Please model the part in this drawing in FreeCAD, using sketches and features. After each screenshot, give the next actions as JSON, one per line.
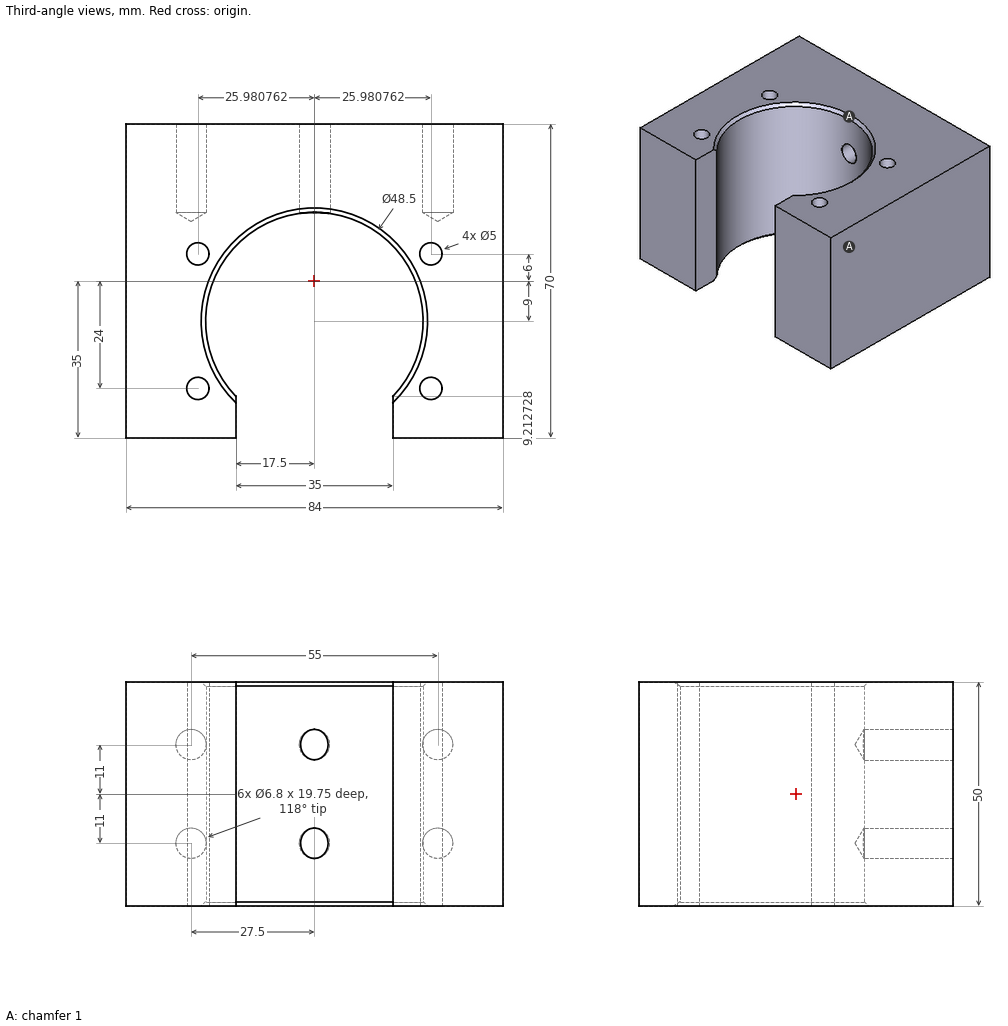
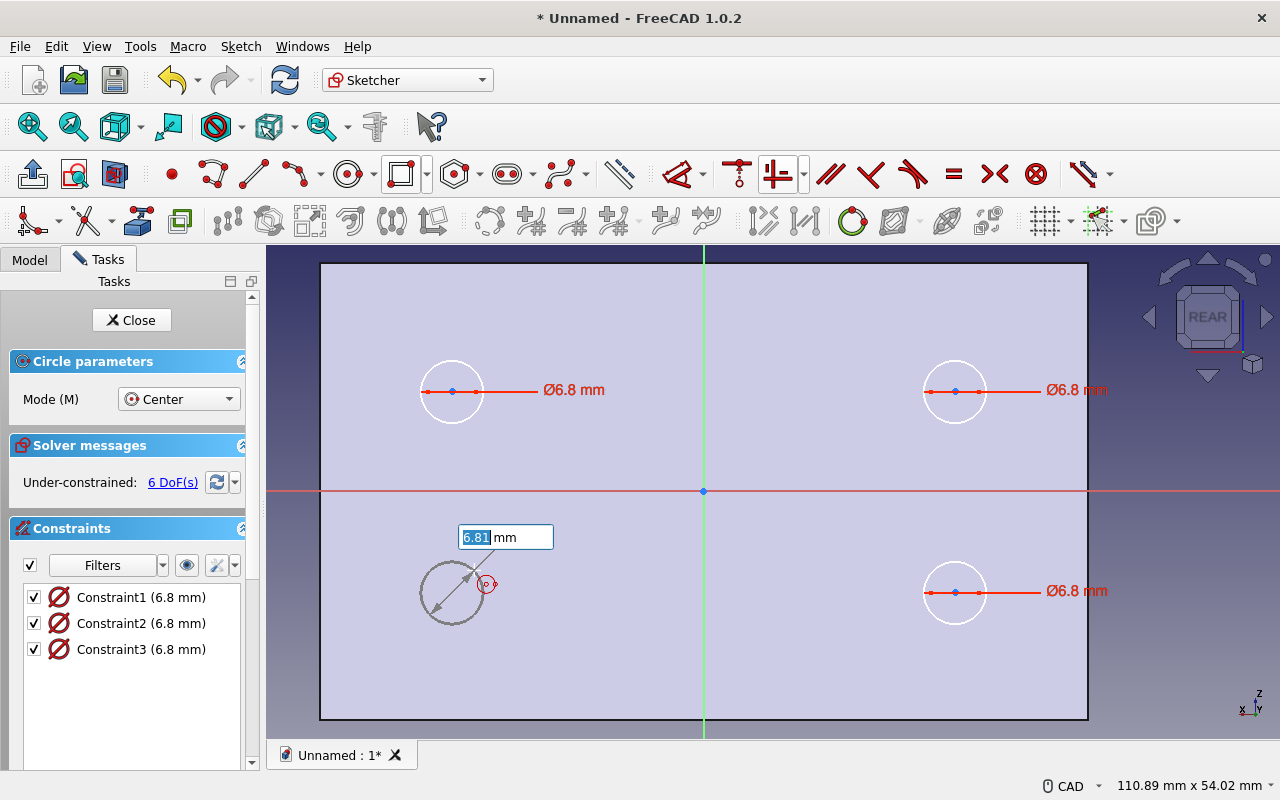
{"action": "type", "text": "6.8"}
{"action": "key", "text": "Return"}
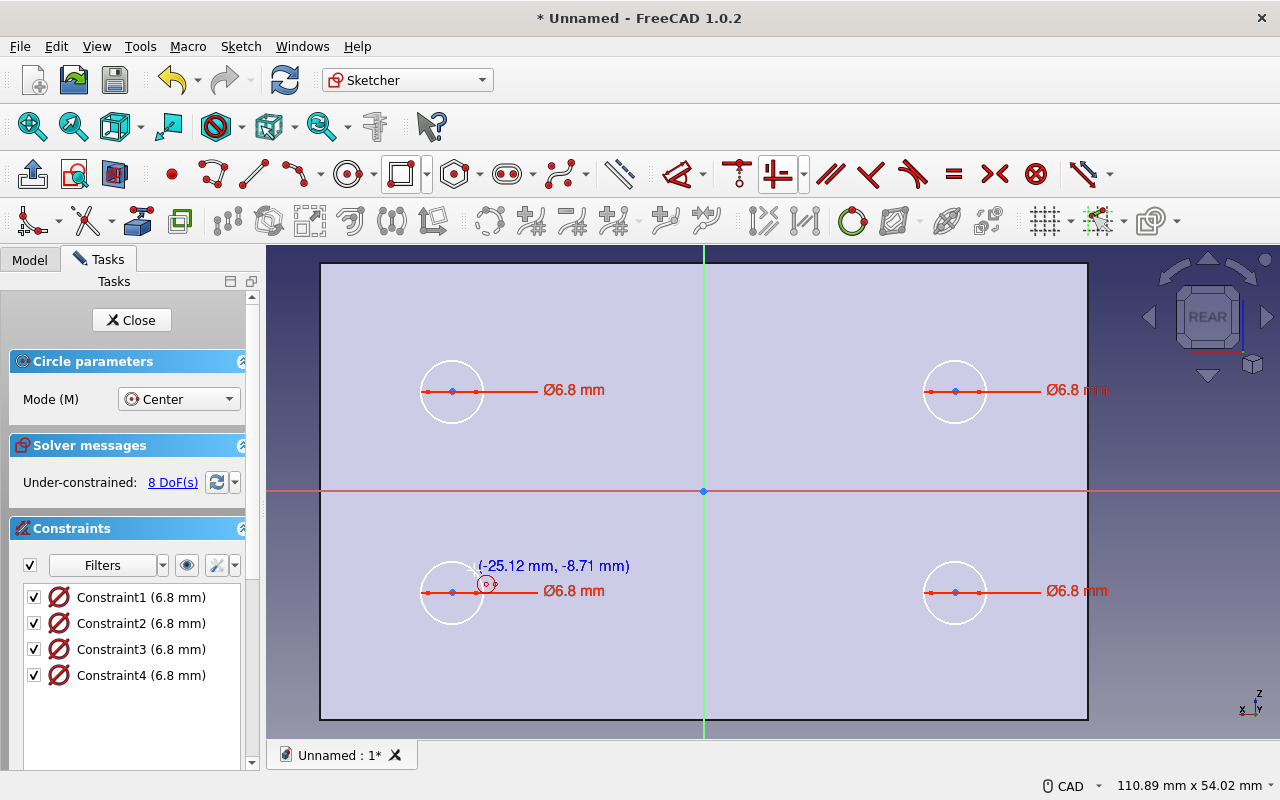
{"action": "left_click", "coordinate": [704, 592]}
{"action": "mouse_move", "coordinate": [726, 570]}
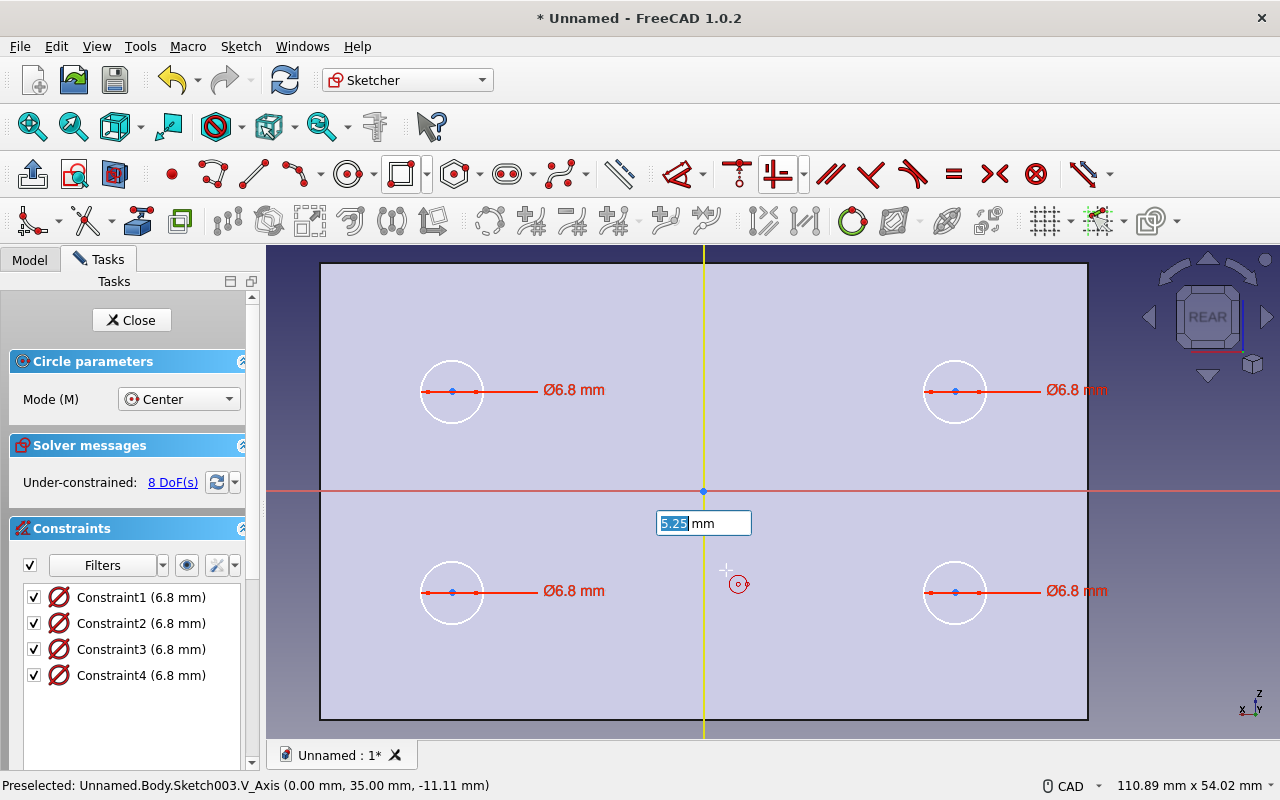
{"action": "type", "text": "6.8"}
{"action": "key", "text": "Return"}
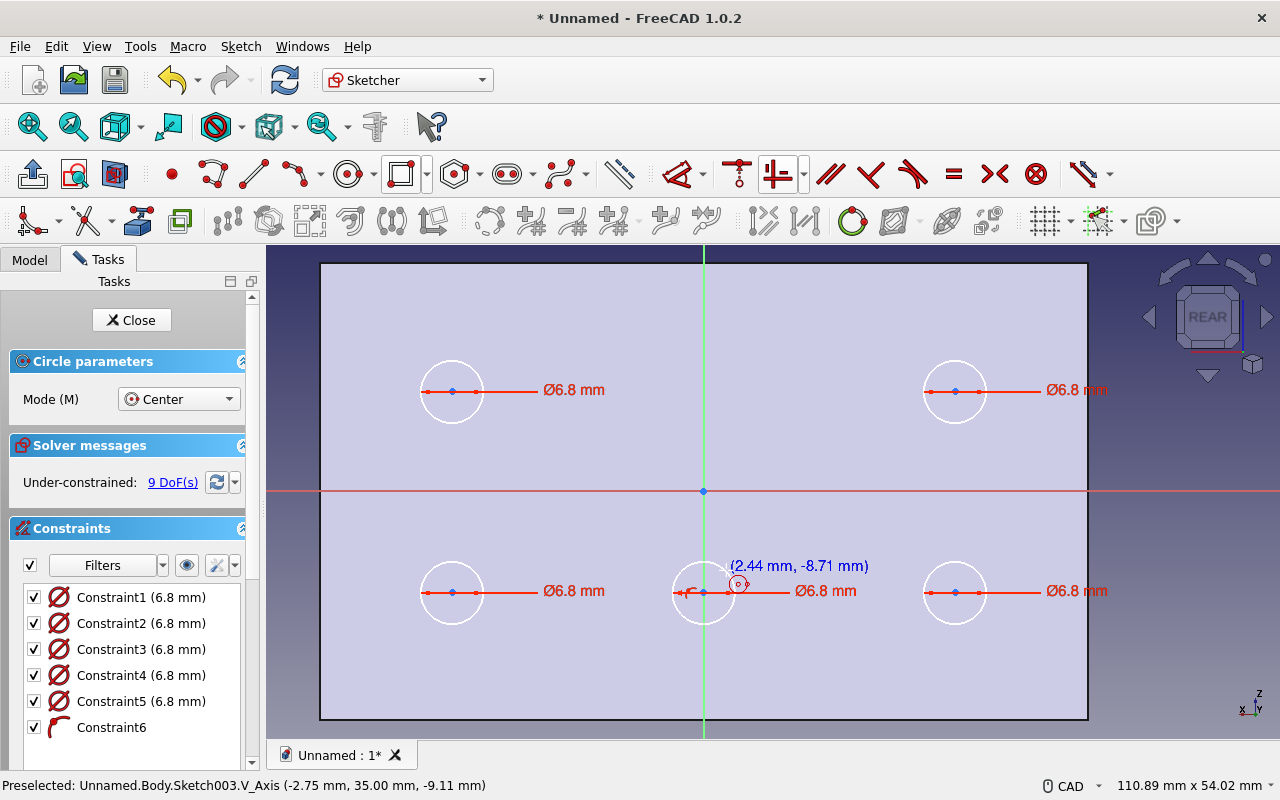
{"action": "left_click", "coordinate": [704, 391]}
{"action": "mouse_move", "coordinate": [726, 369]}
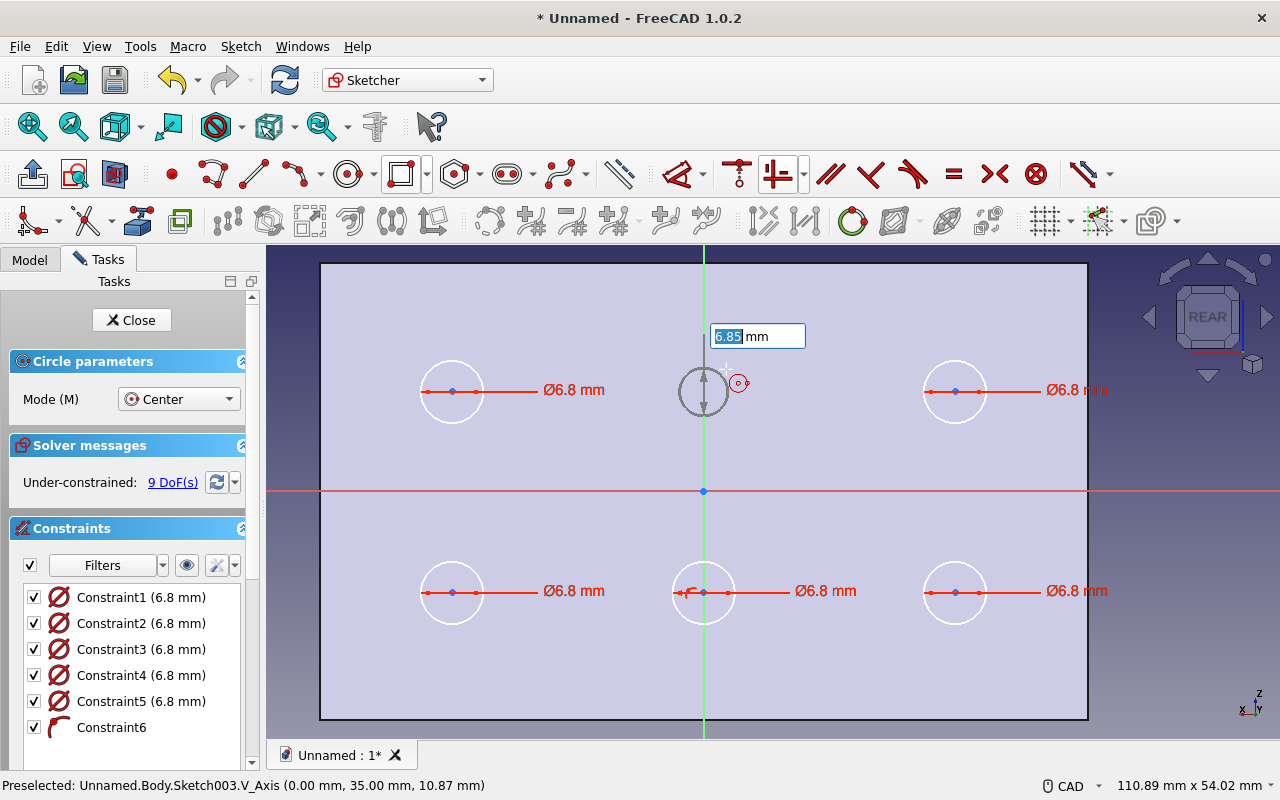
{"action": "type", "text": "6.8"}
{"action": "key", "text": "Return"}
{"action": "key", "text": "Escape"}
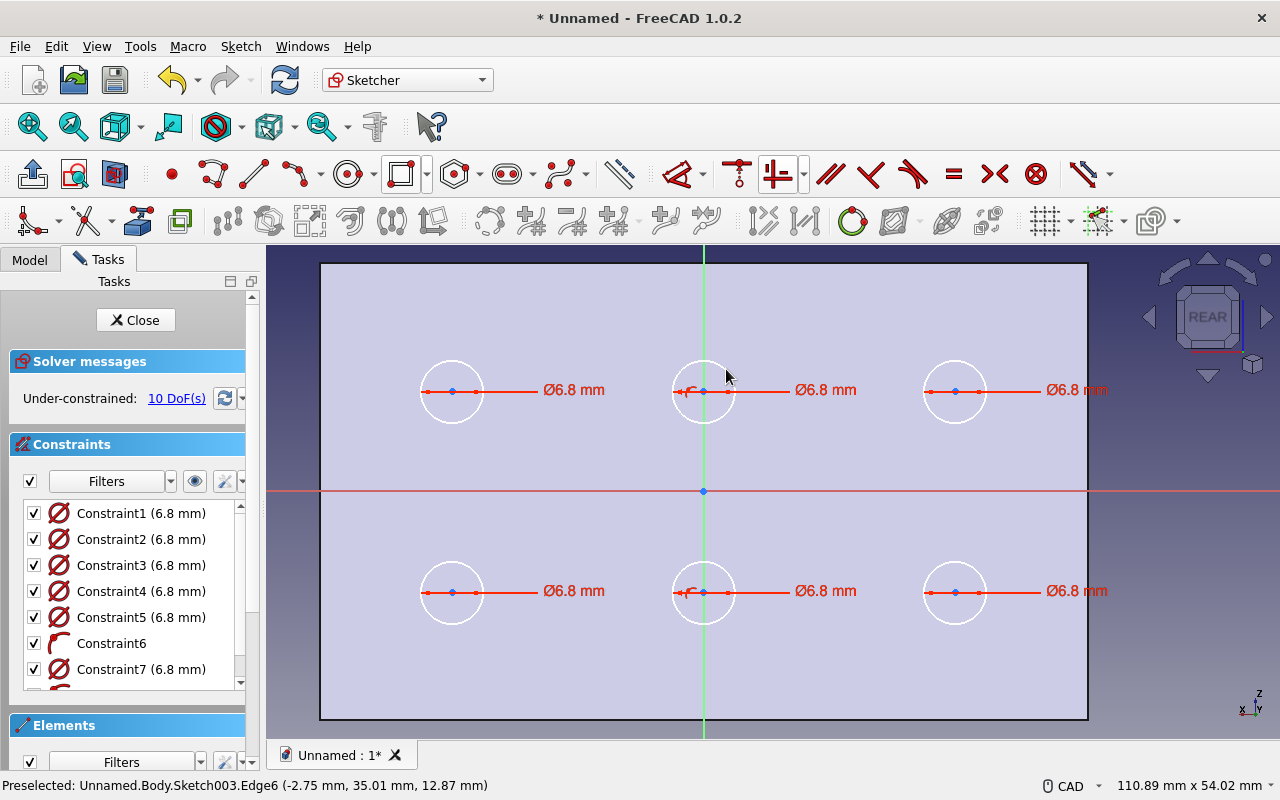
{"action": "left_click", "coordinate": [955, 593]}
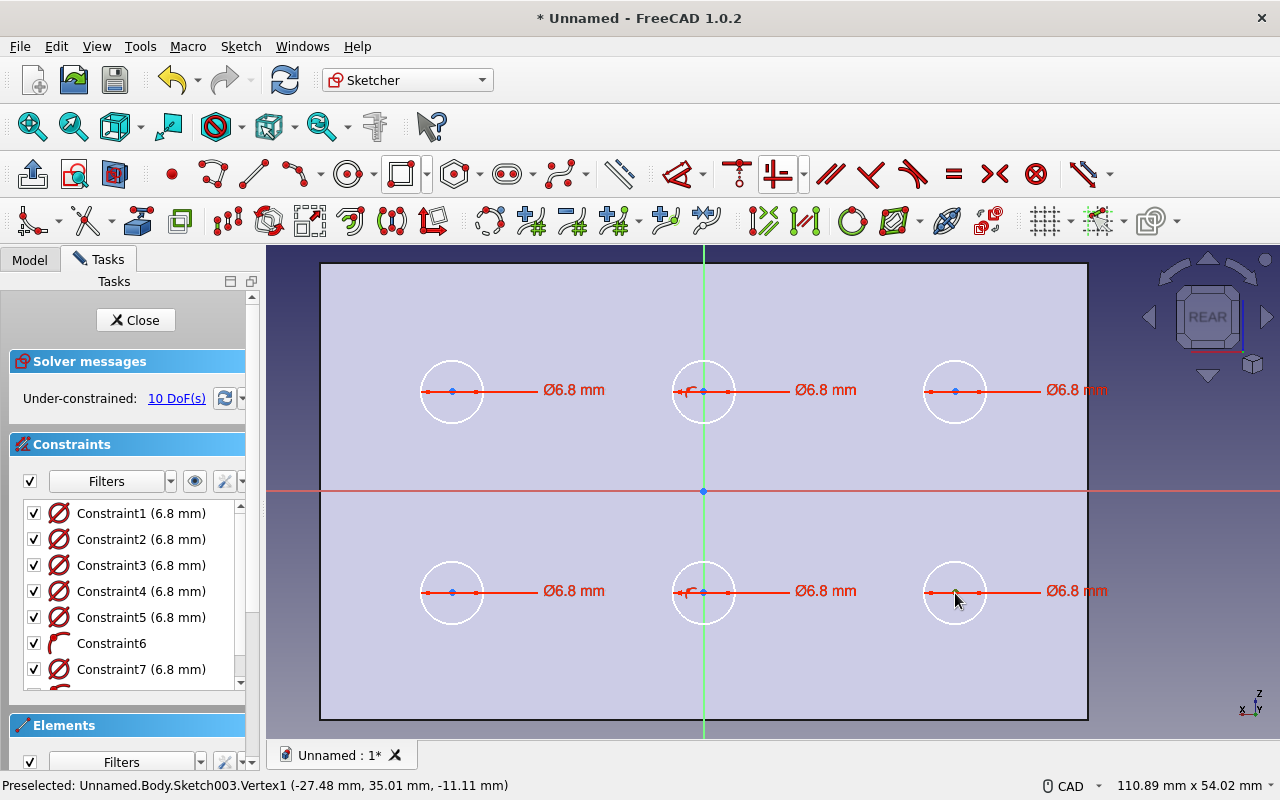
{"action": "left_click", "coordinate": [955, 392]}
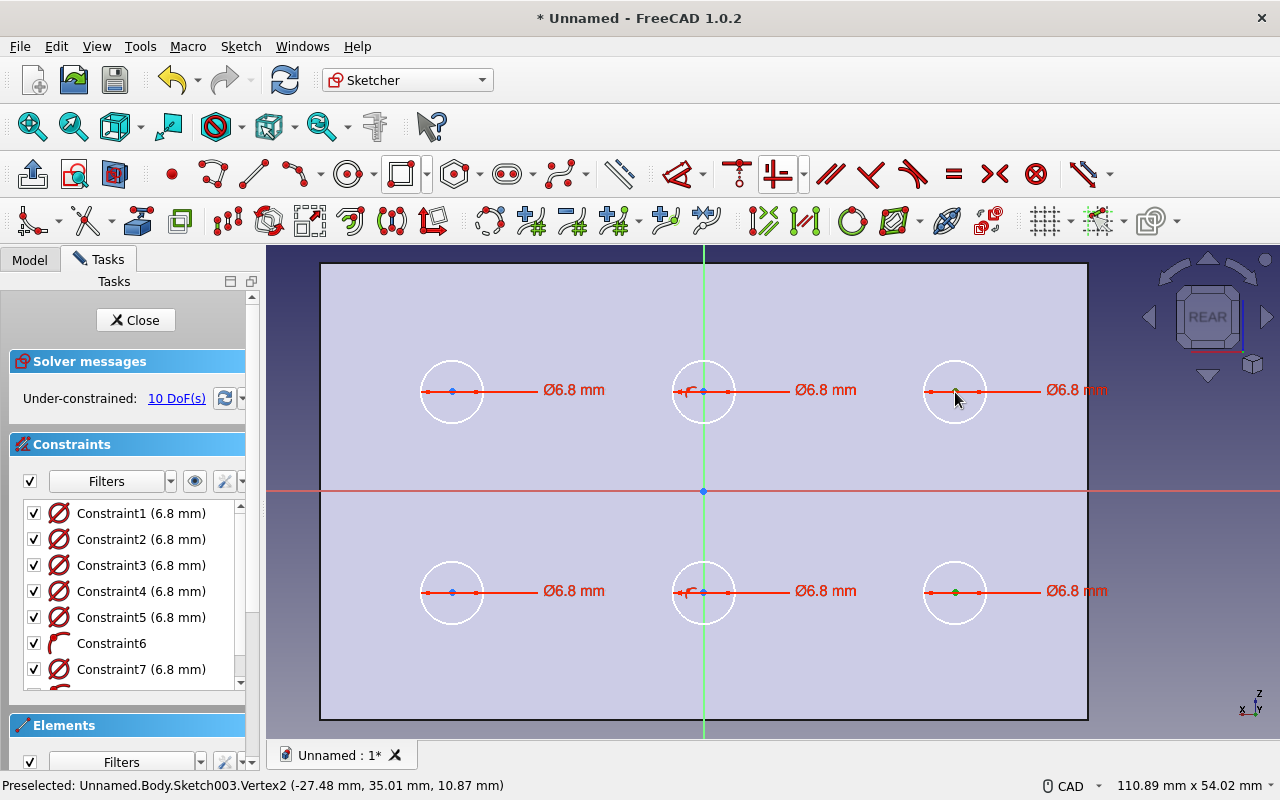
{"action": "key", "text": "v"}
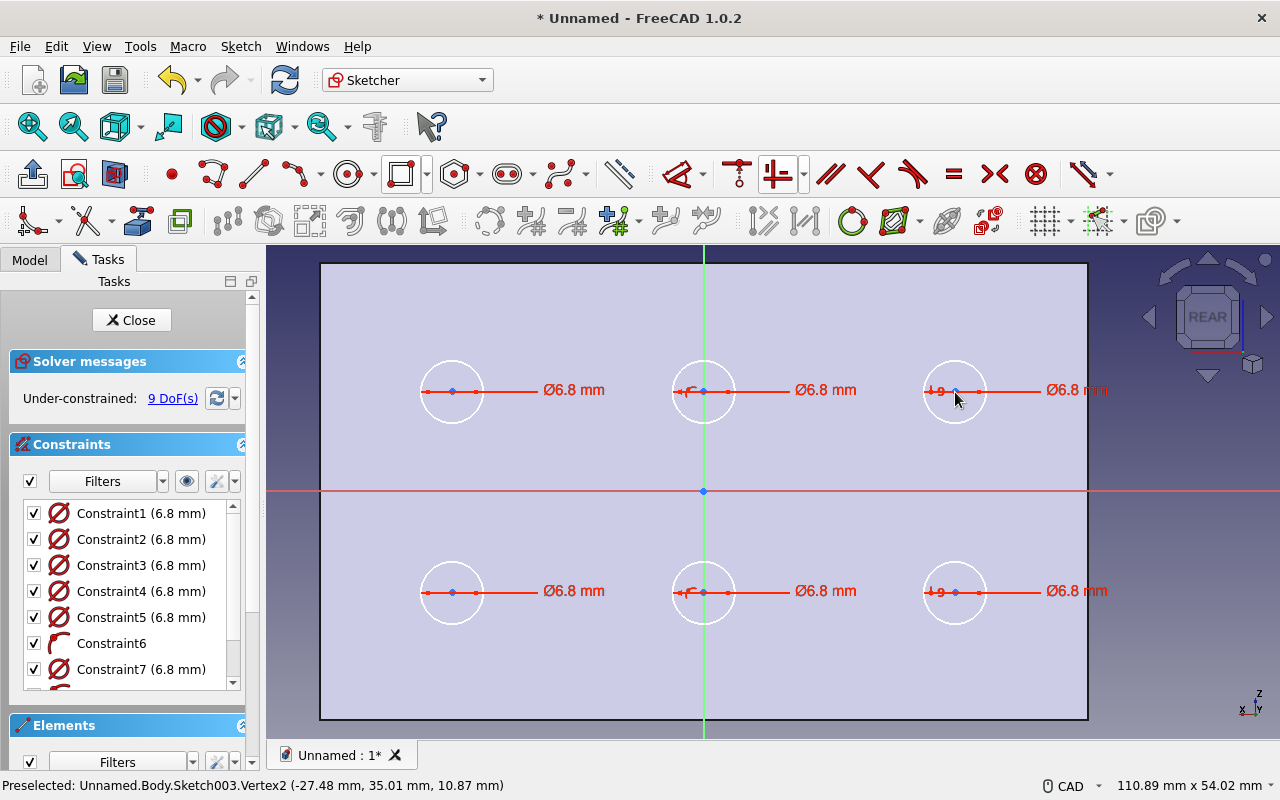
{"action": "left_click", "coordinate": [955, 392]}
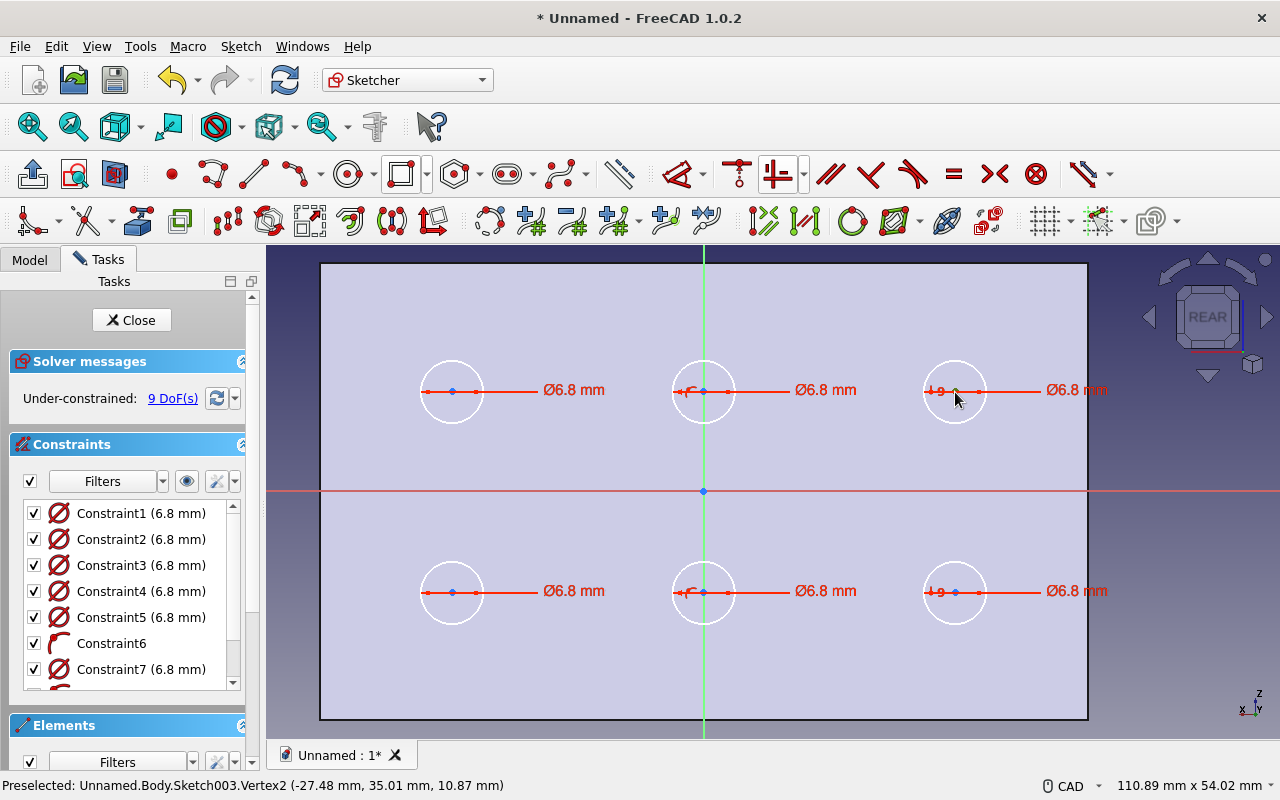
{"action": "left_click", "coordinate": [452, 392]}